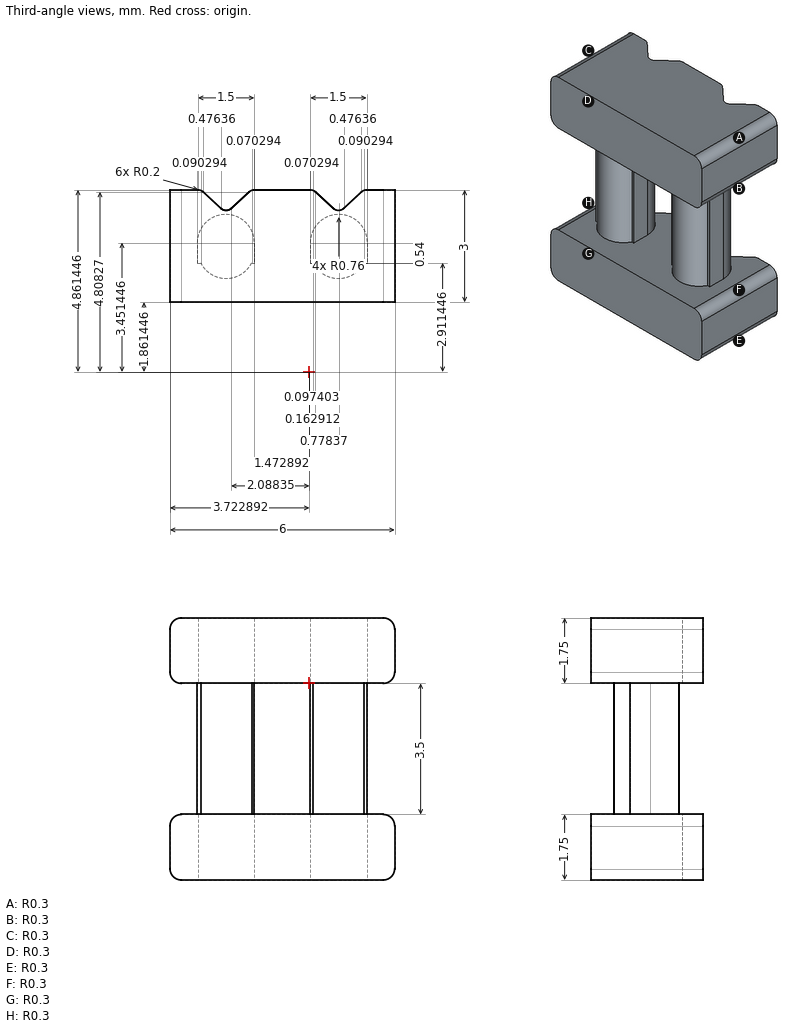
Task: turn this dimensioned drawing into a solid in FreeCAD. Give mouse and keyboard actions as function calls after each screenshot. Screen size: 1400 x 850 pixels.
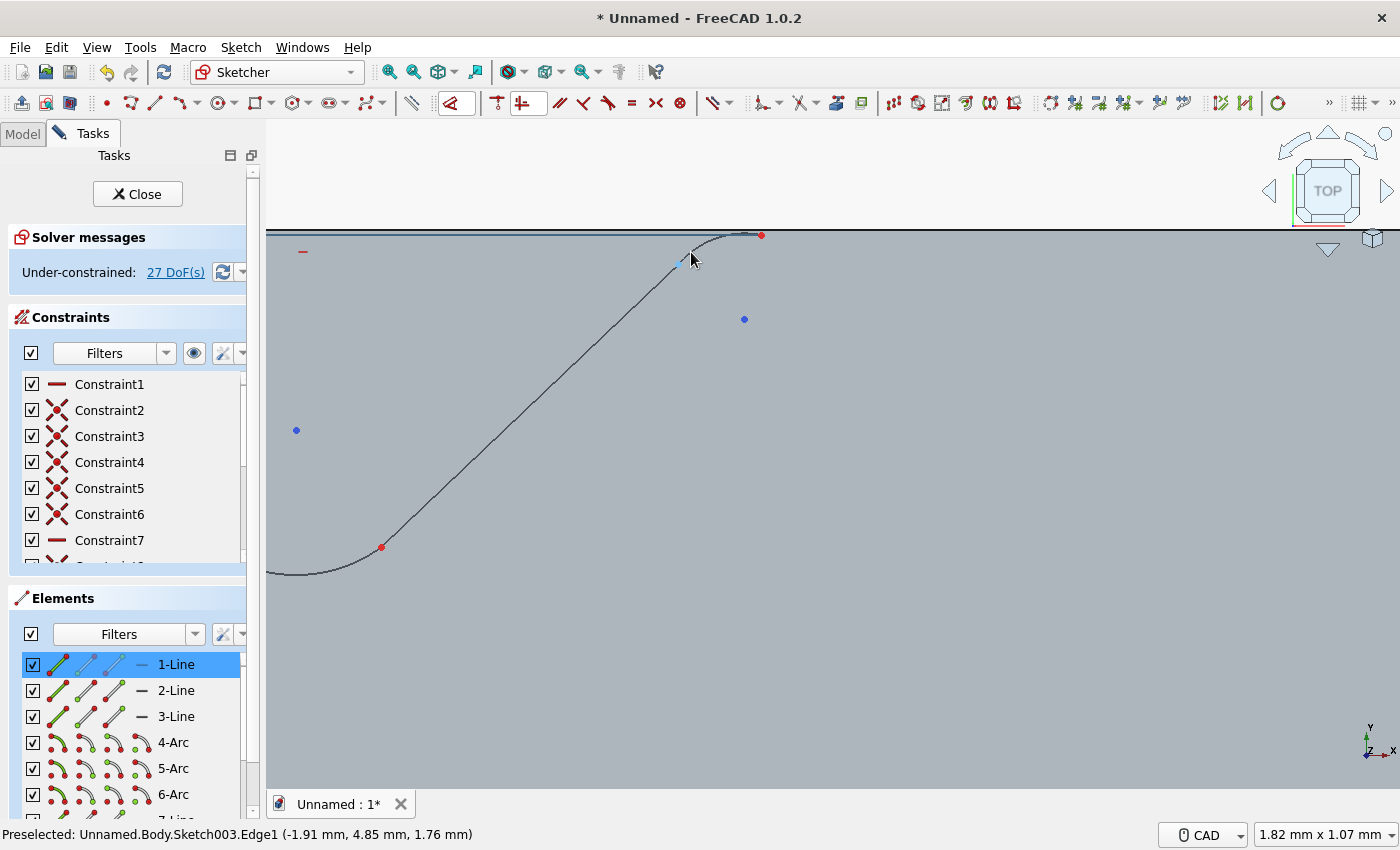
click(692, 252)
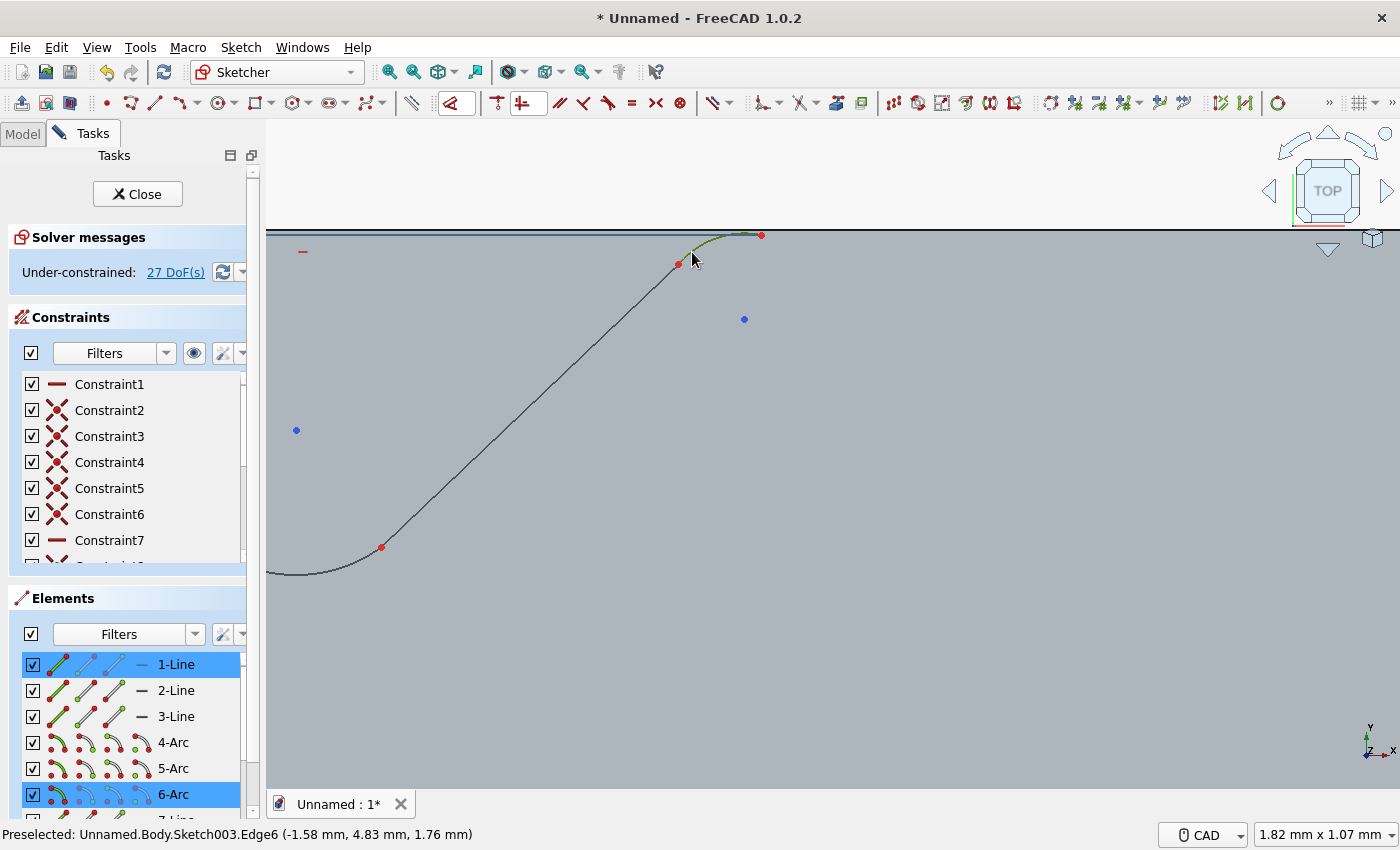
click(608, 104)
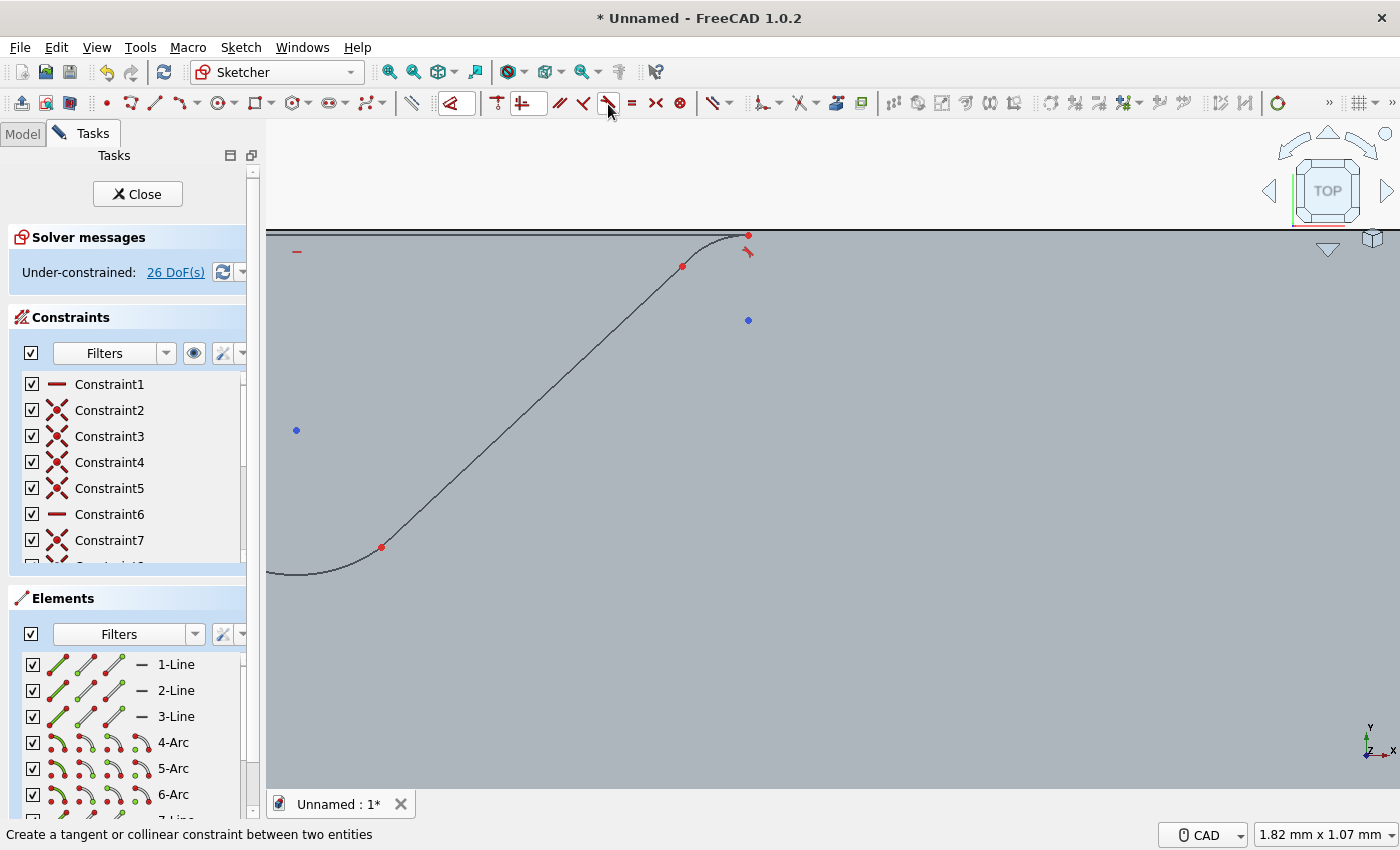
scroll(692, 252, down, 10)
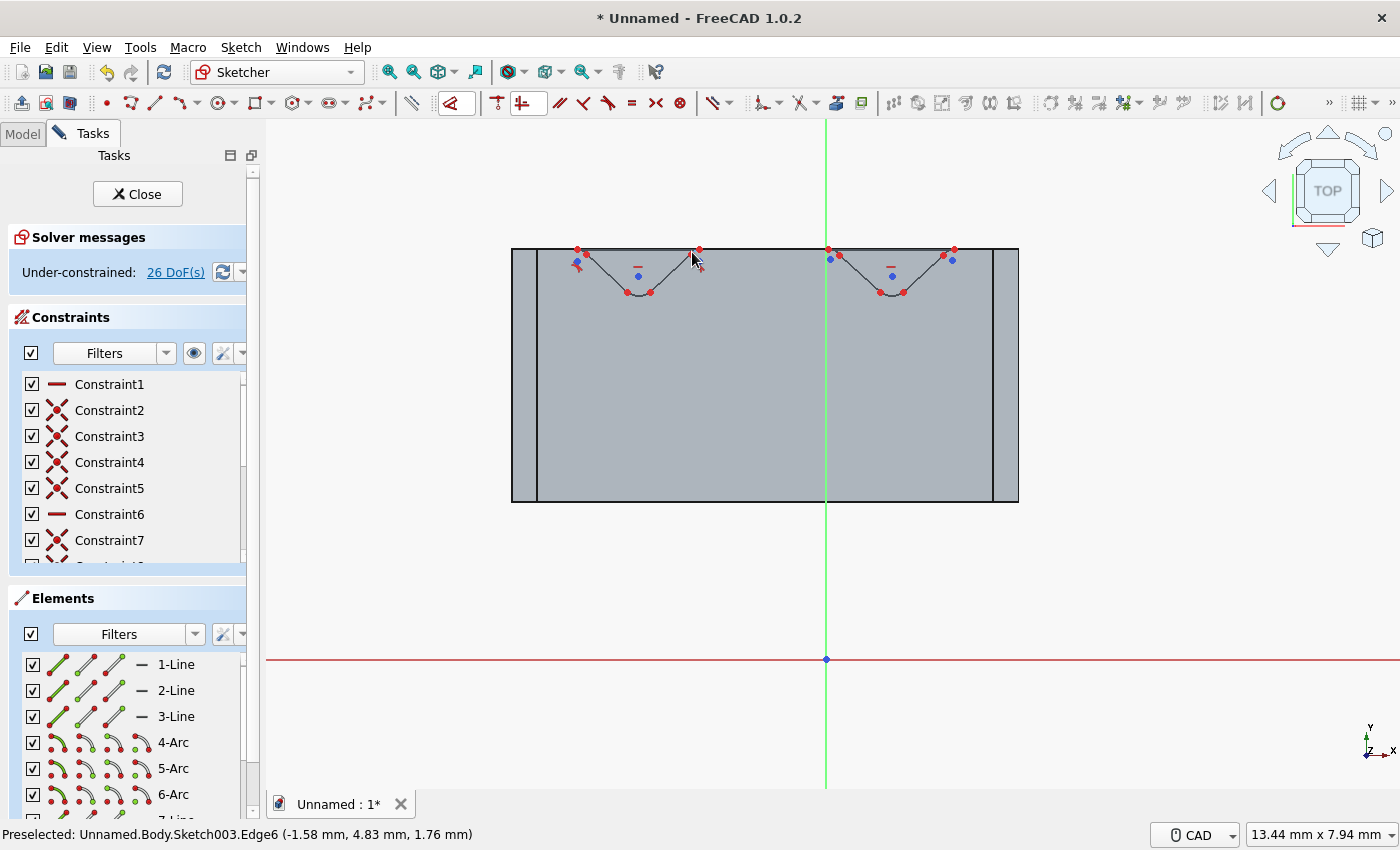
click(599, 265)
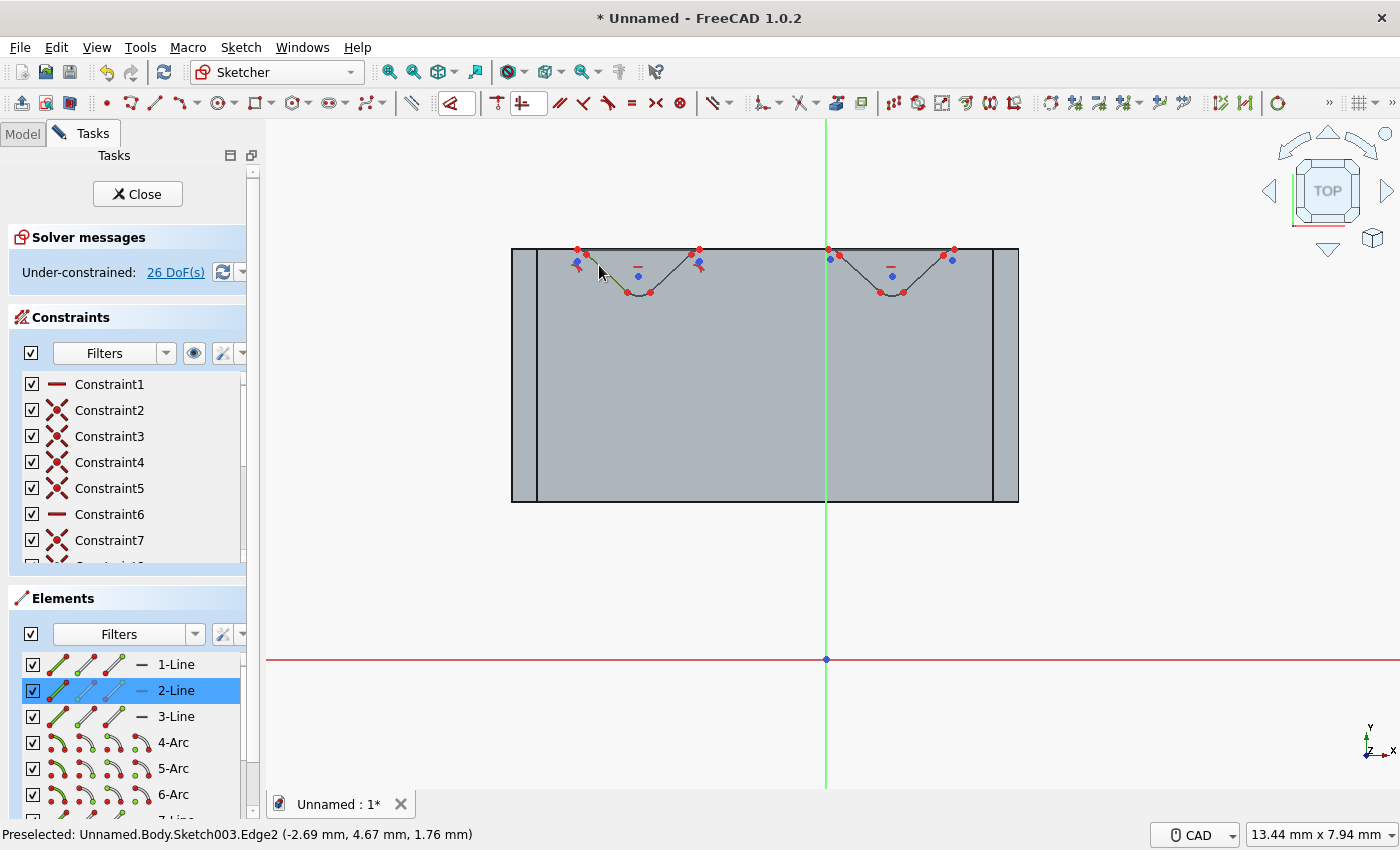
scroll(585, 252, up, 10)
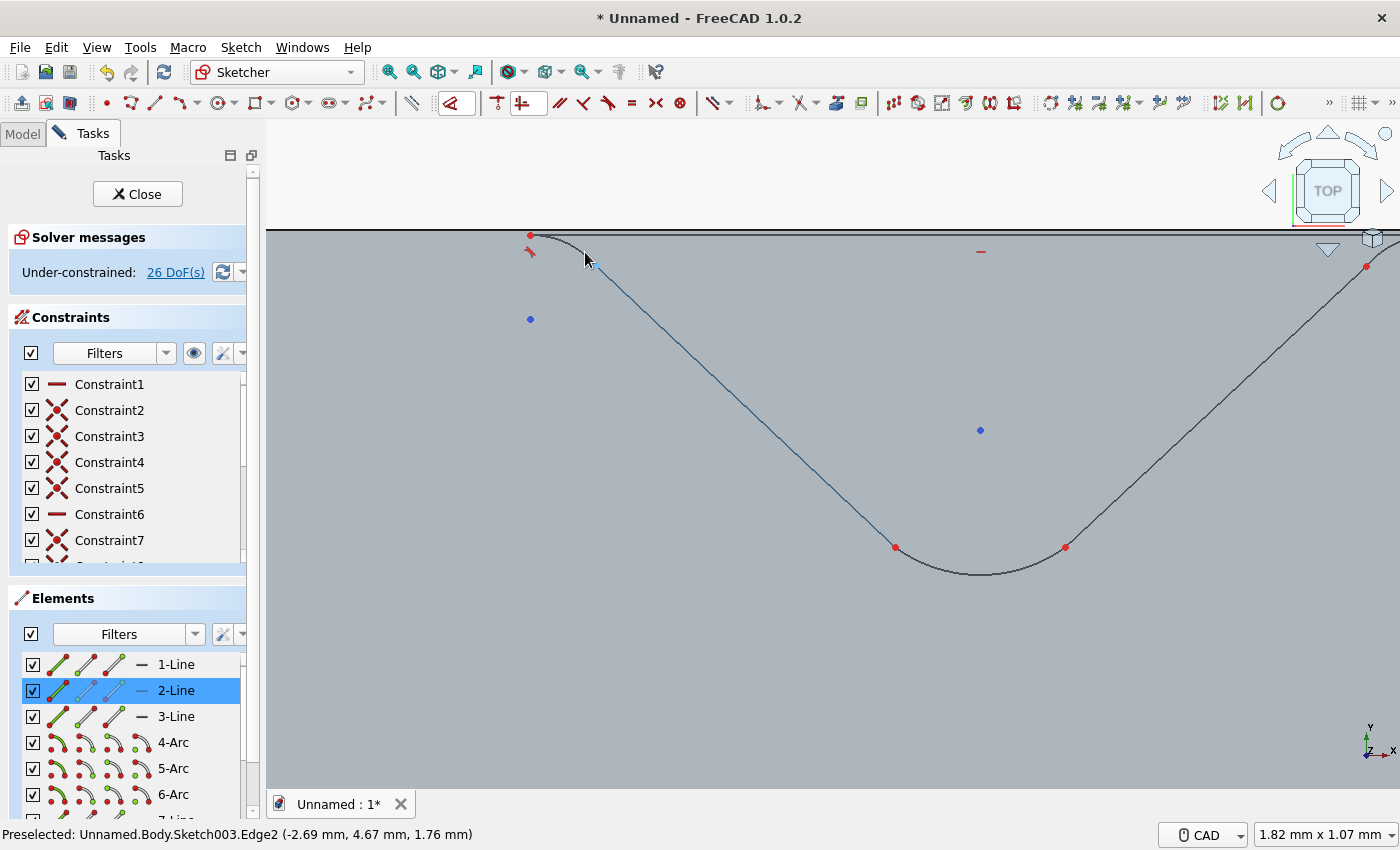
click(580, 251)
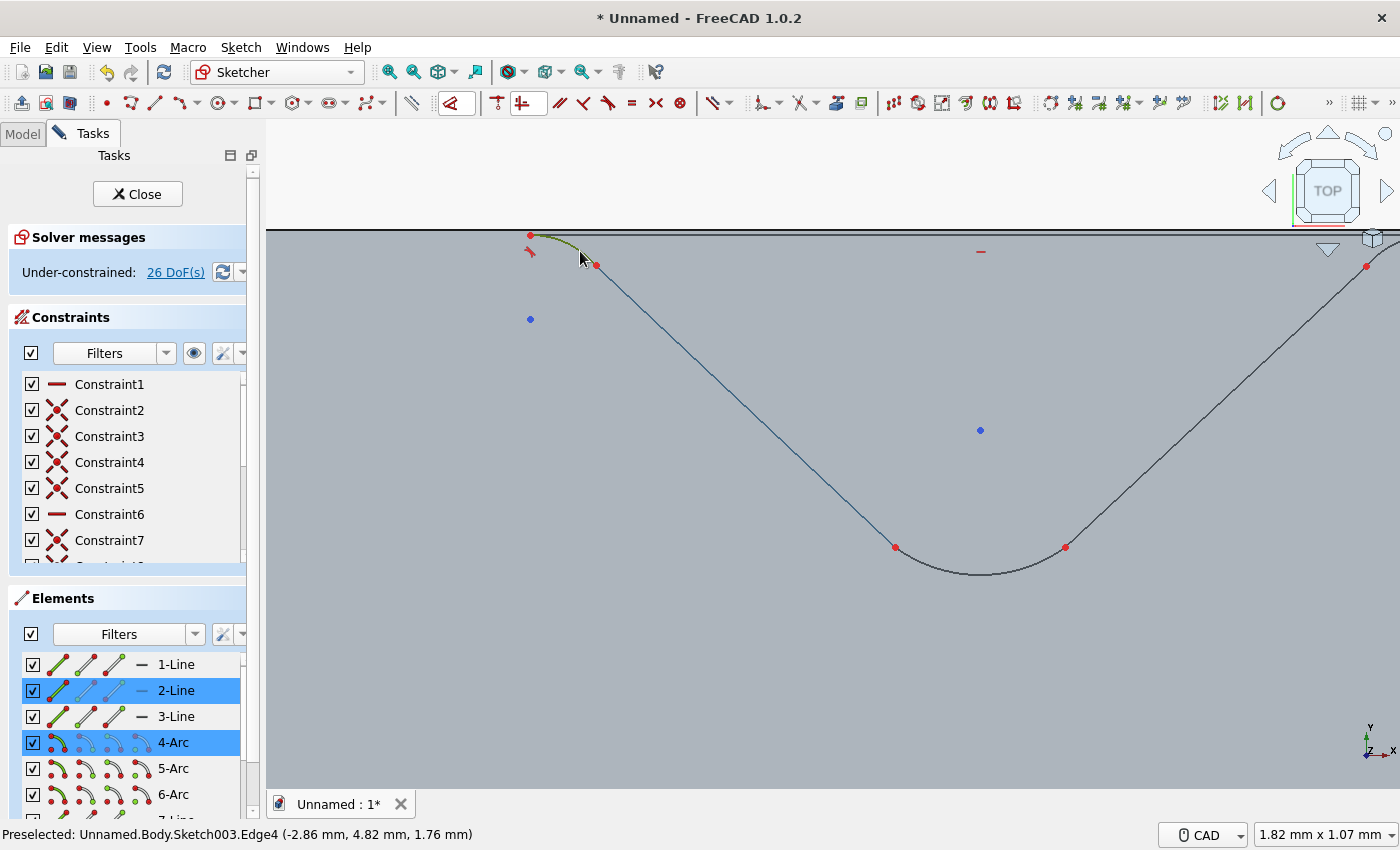
click(608, 104)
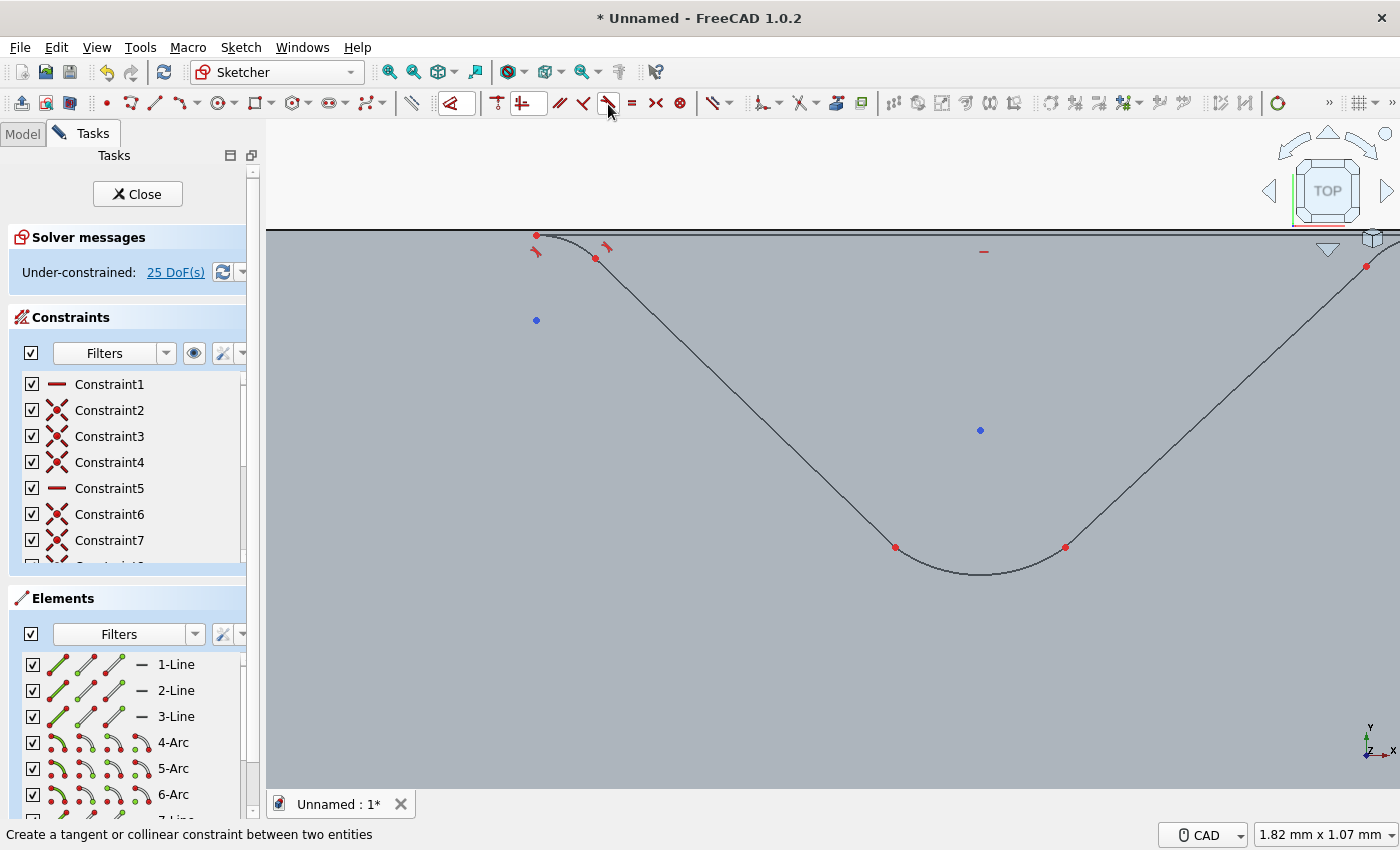
scroll(584, 252, down, 10)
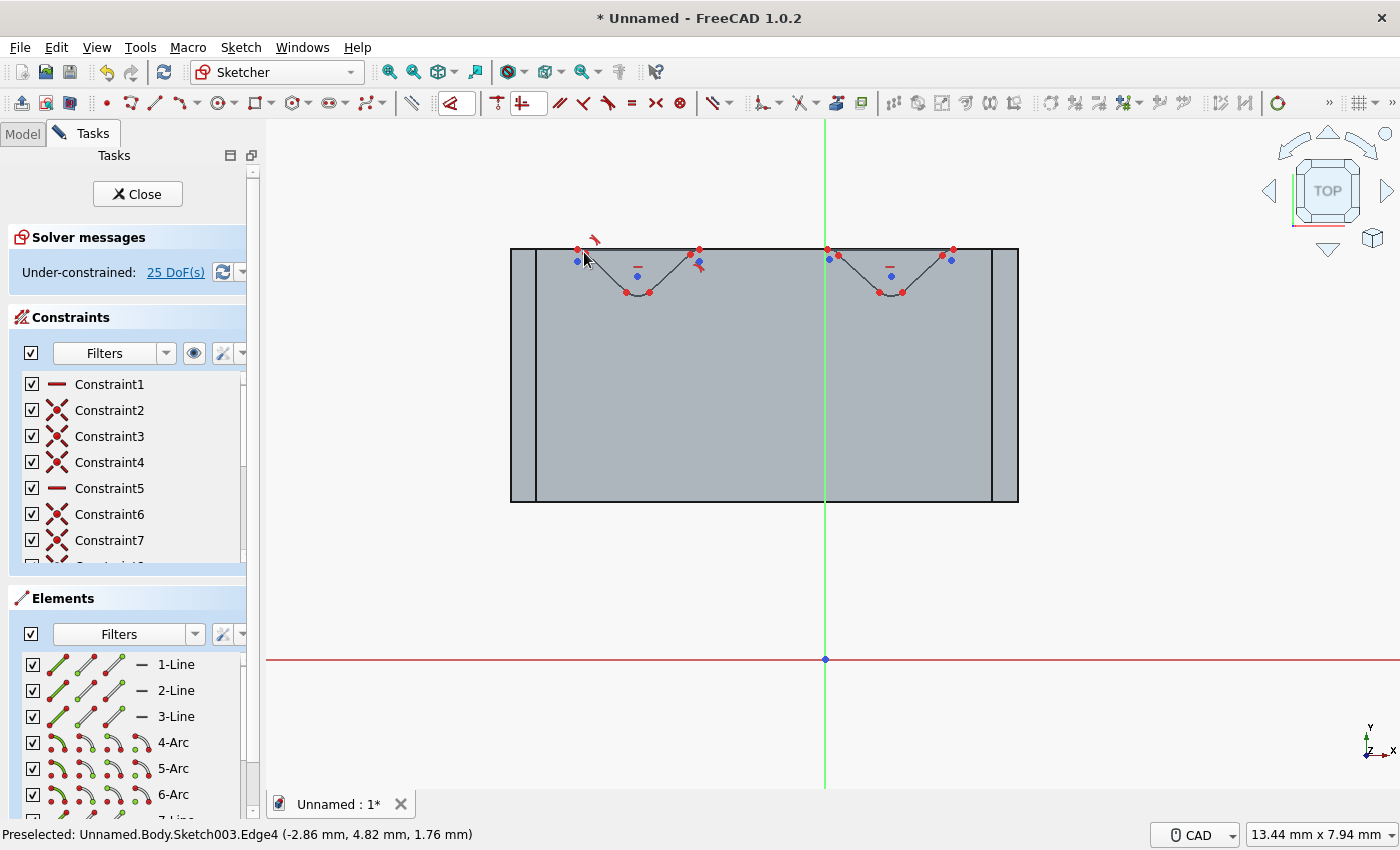
click(598, 265)